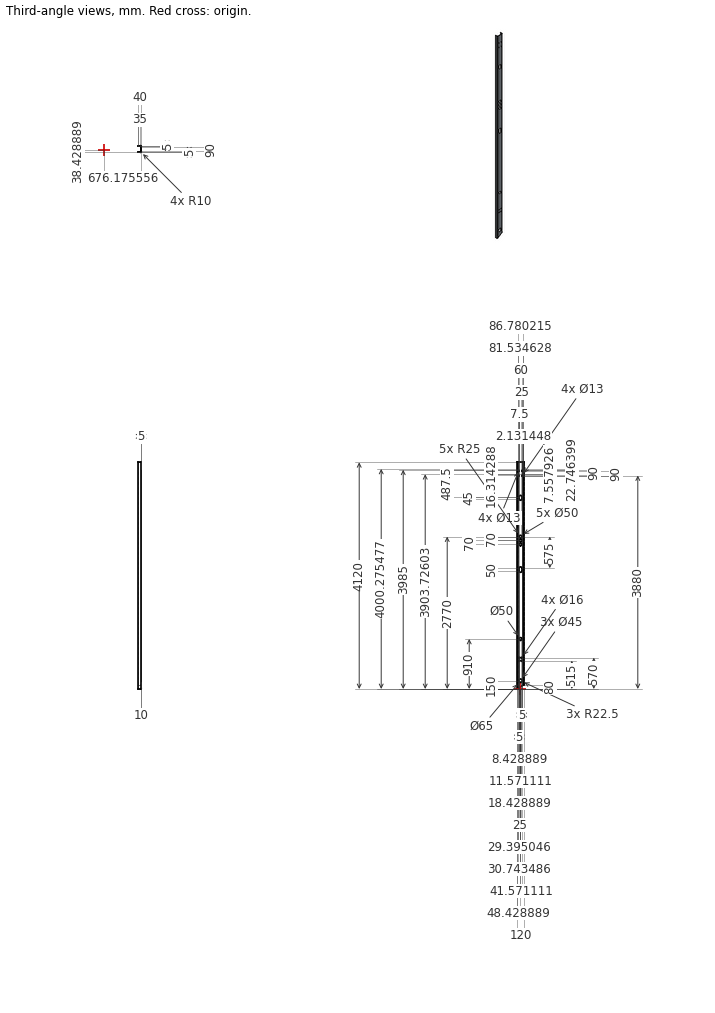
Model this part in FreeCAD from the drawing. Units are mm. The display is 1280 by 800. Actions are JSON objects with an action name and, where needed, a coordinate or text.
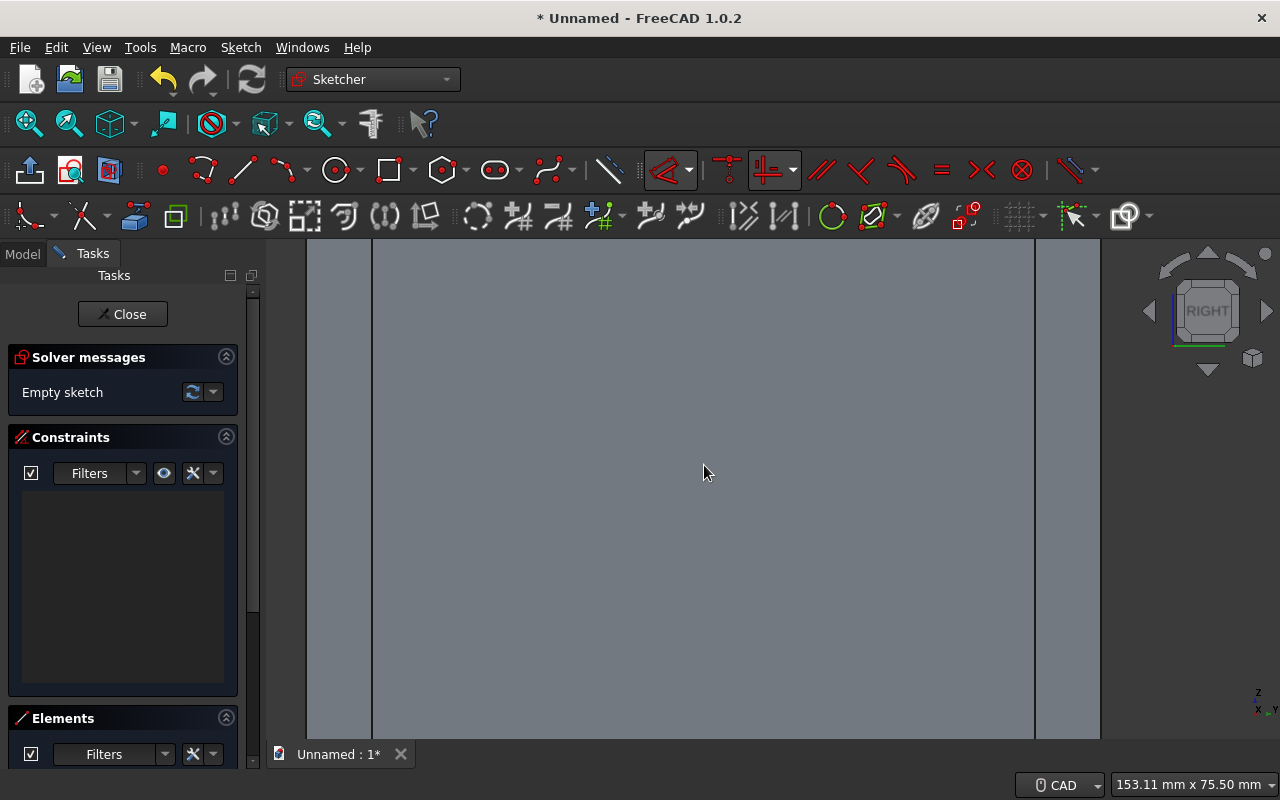
{"action": "left_click", "coordinate": [336, 170]}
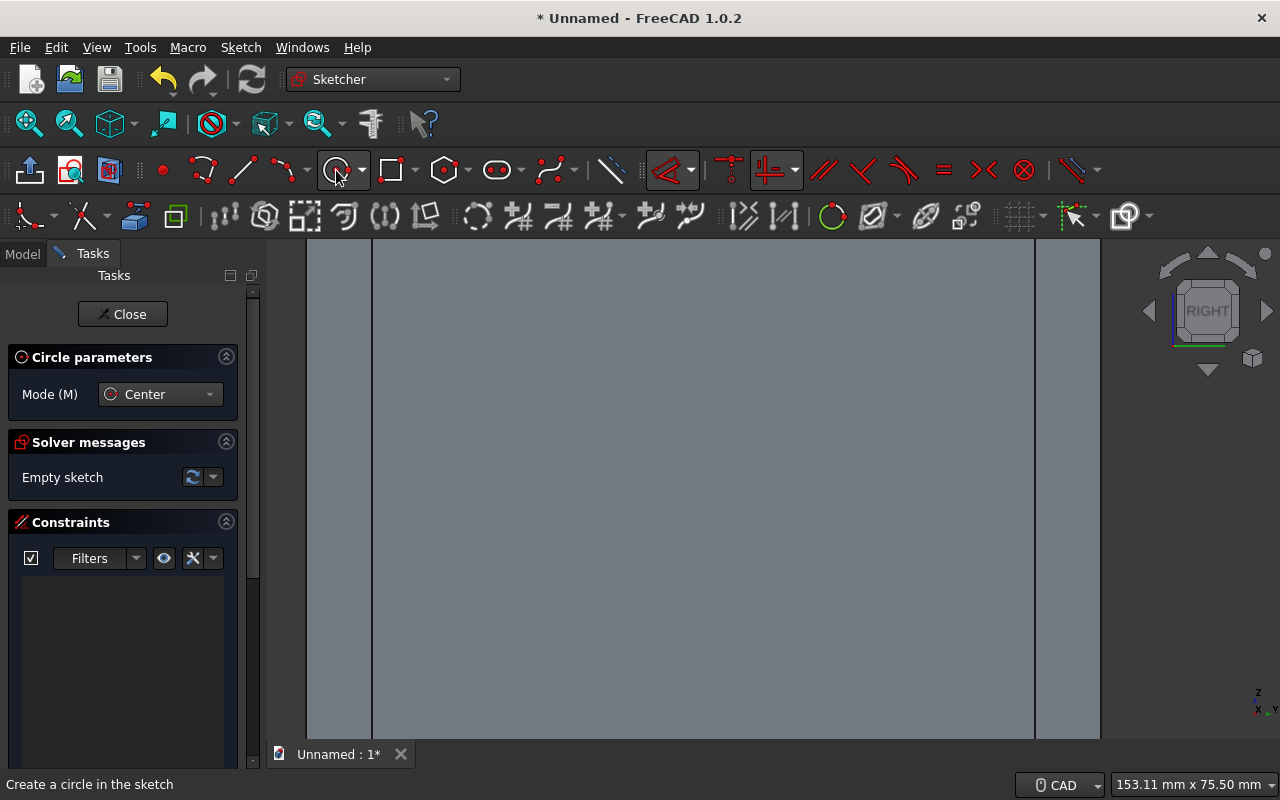
{"action": "left_click", "coordinate": [703, 488]}
{"action": "mouse_move", "coordinate": [821, 370]}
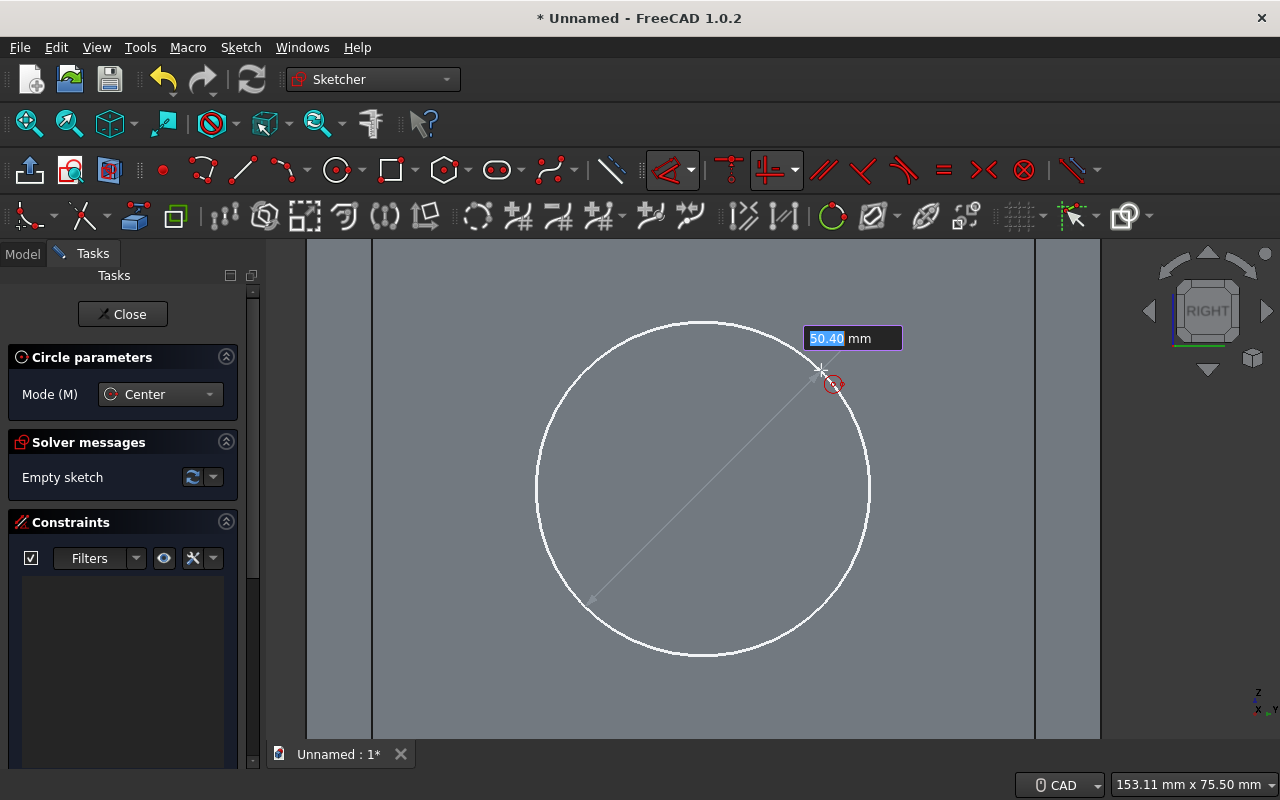
{"action": "type", "text": "50"}
{"action": "key", "text": "Return"}
{"action": "key", "text": "Escape"}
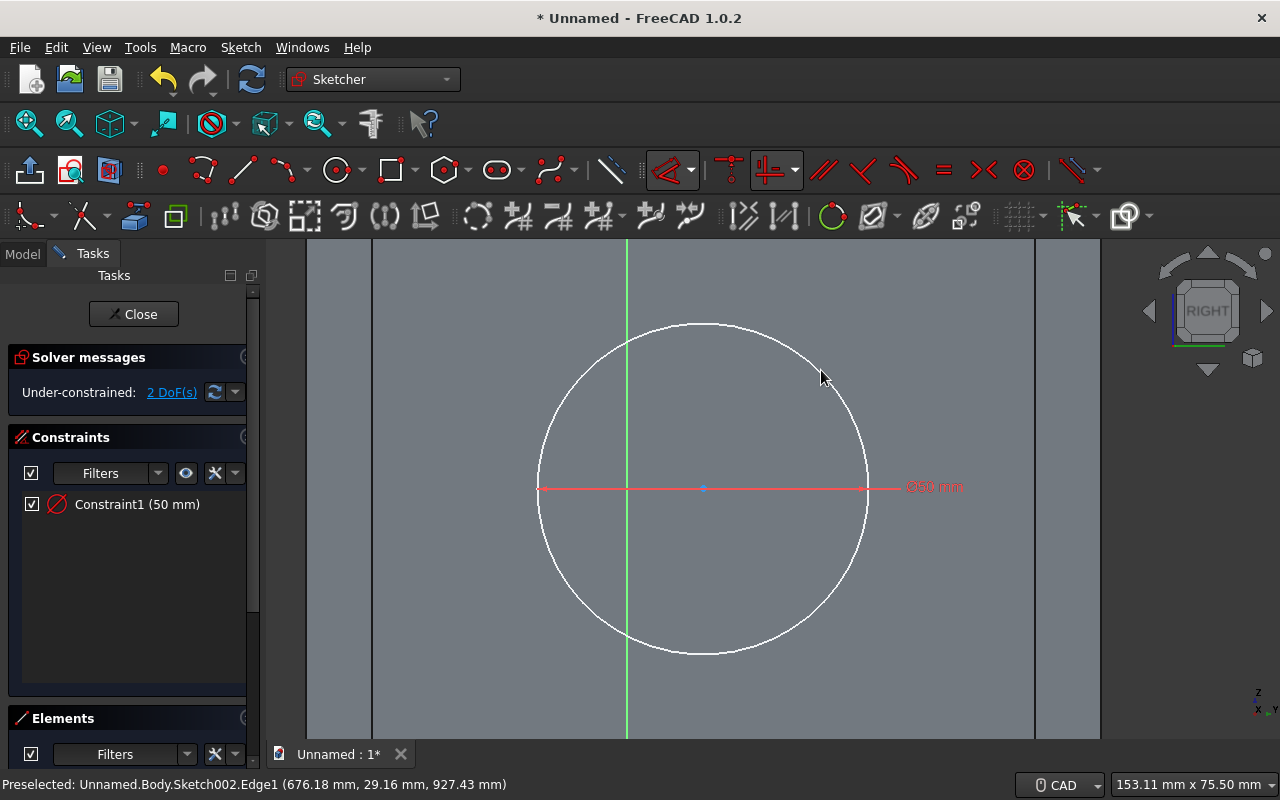
{"action": "left_click", "coordinate": [703, 489]}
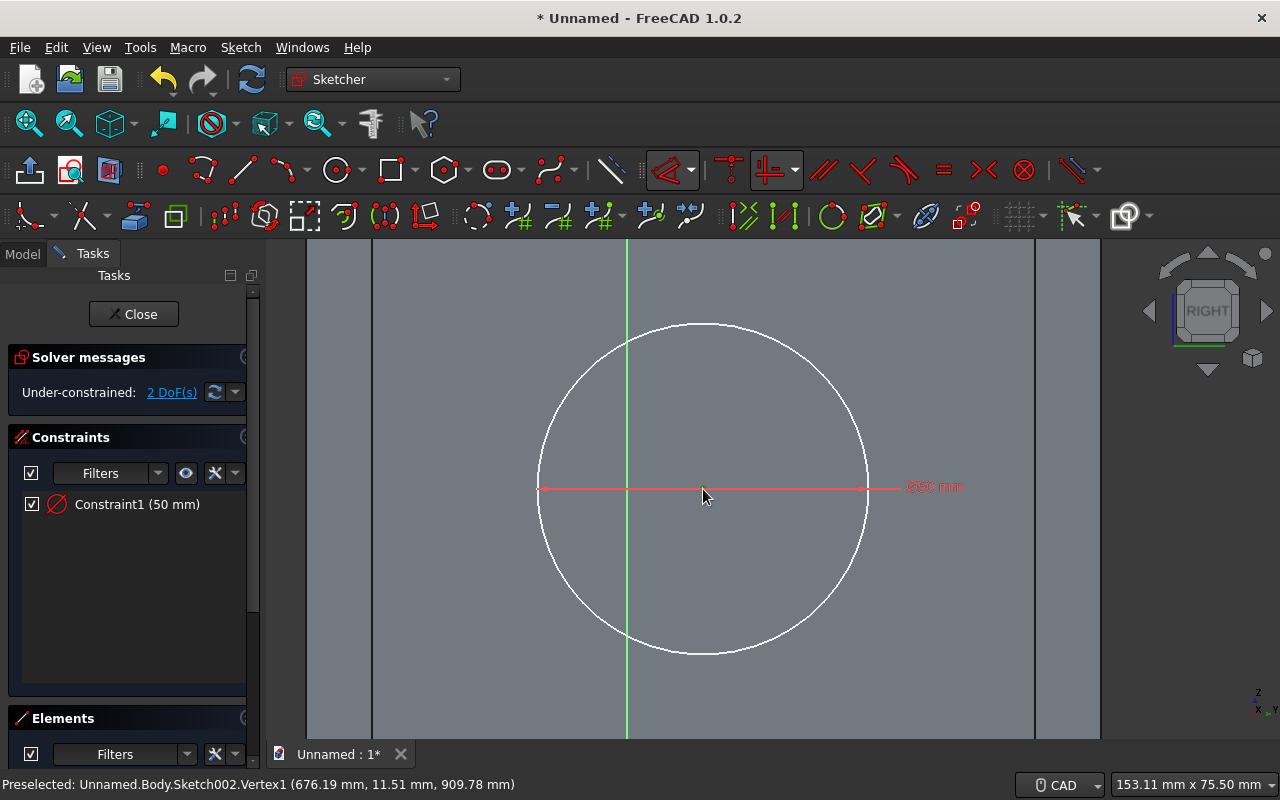
{"action": "key", "text": "i"}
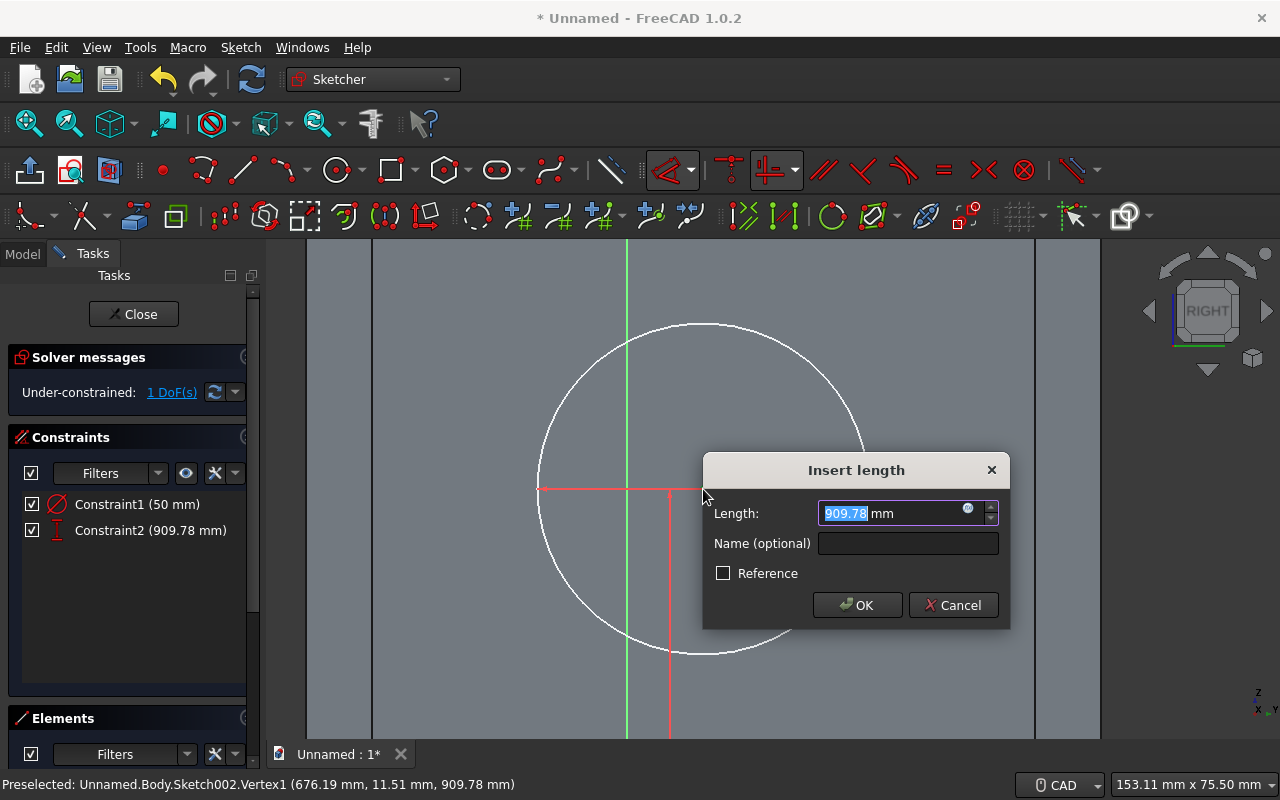
{"action": "type", "text": "910"}
{"action": "key", "text": "Return"}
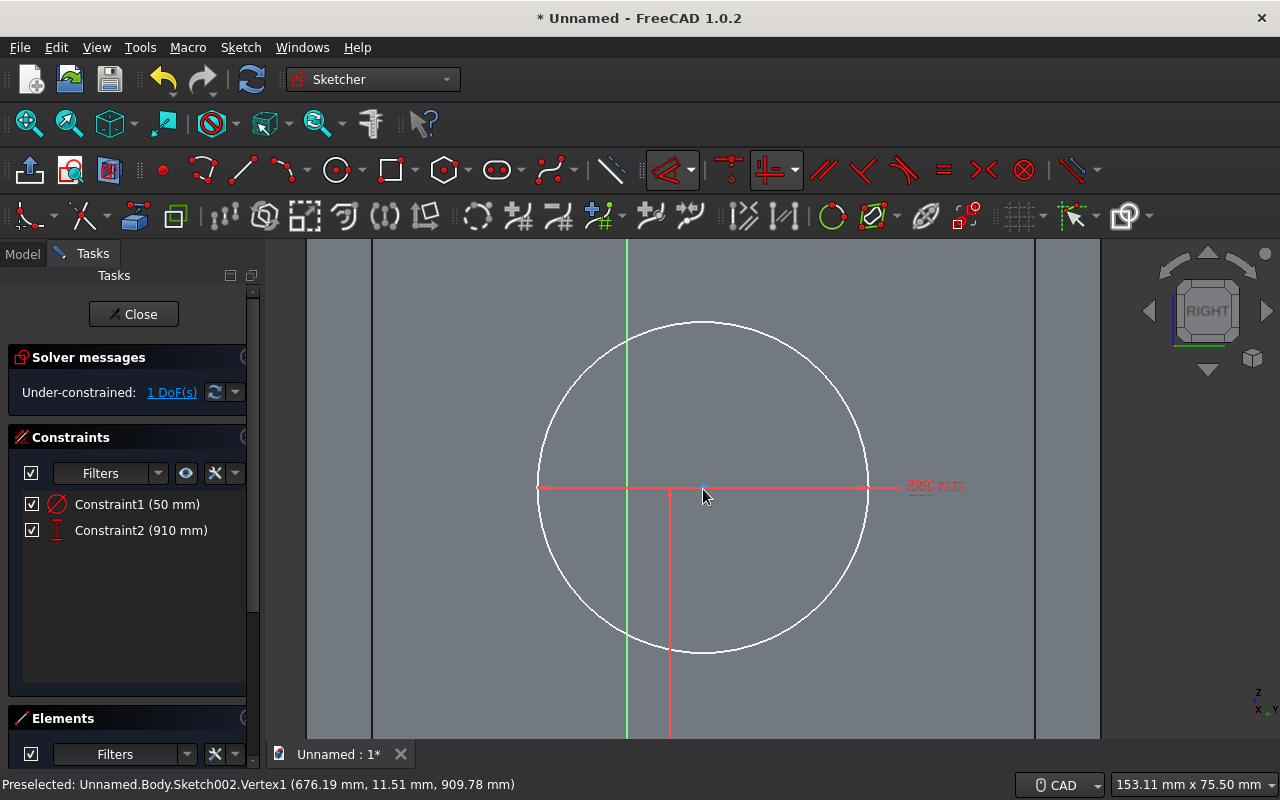
{"action": "left_click", "coordinate": [703, 488]}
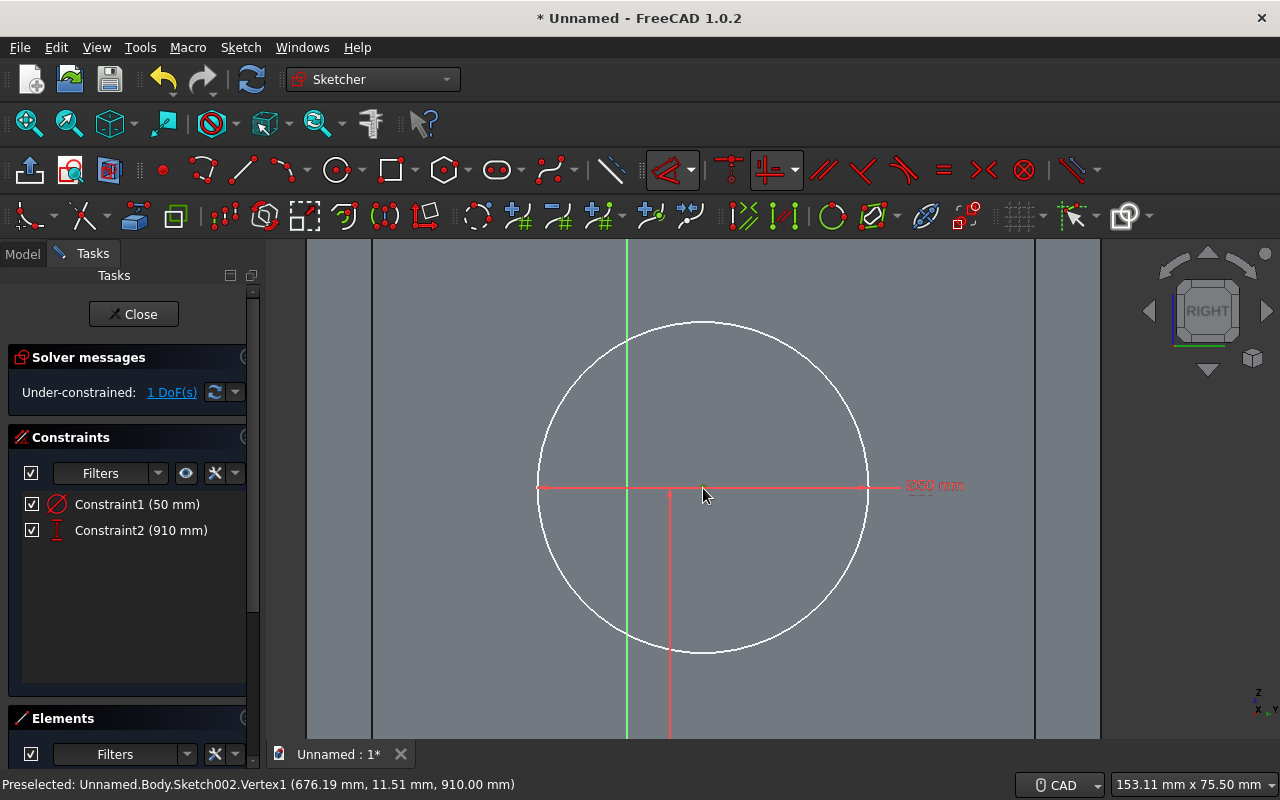
{"action": "left_click", "coordinate": [694, 170]}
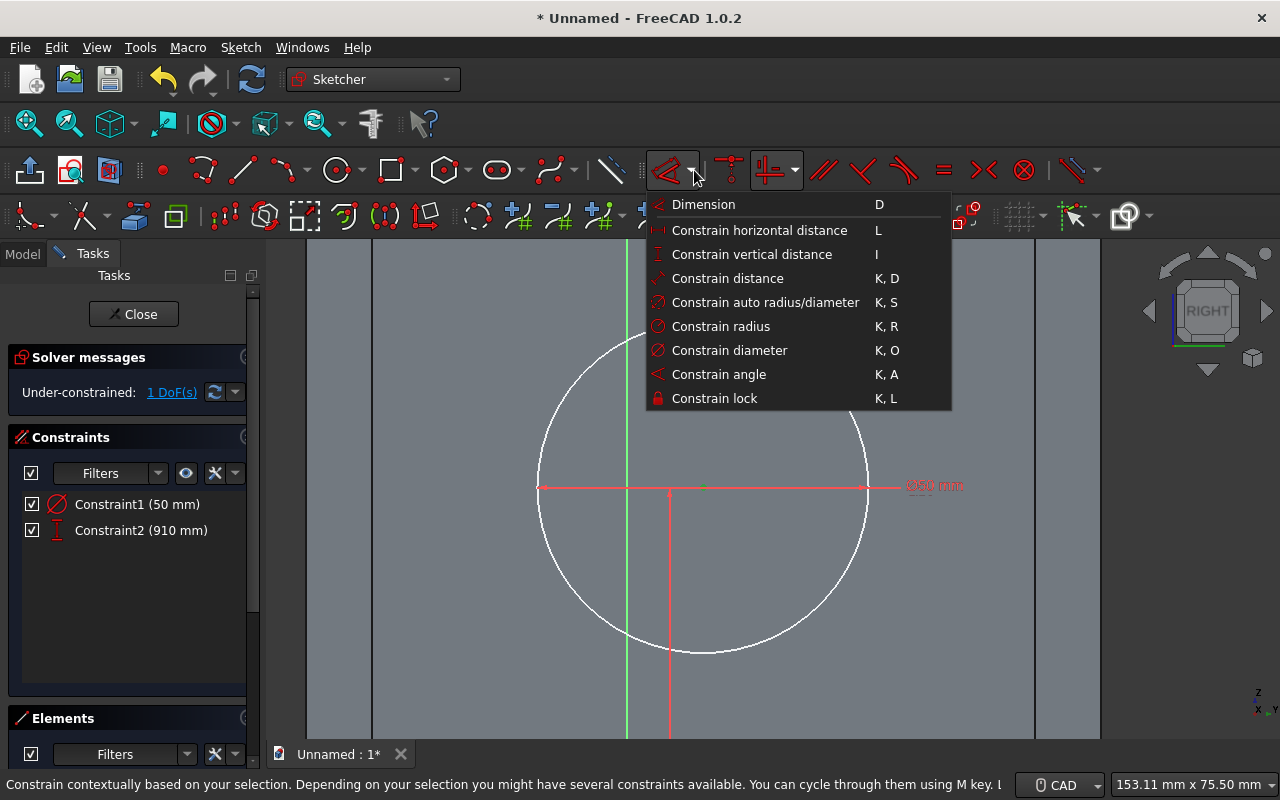
{"action": "left_click", "coordinate": [799, 230]}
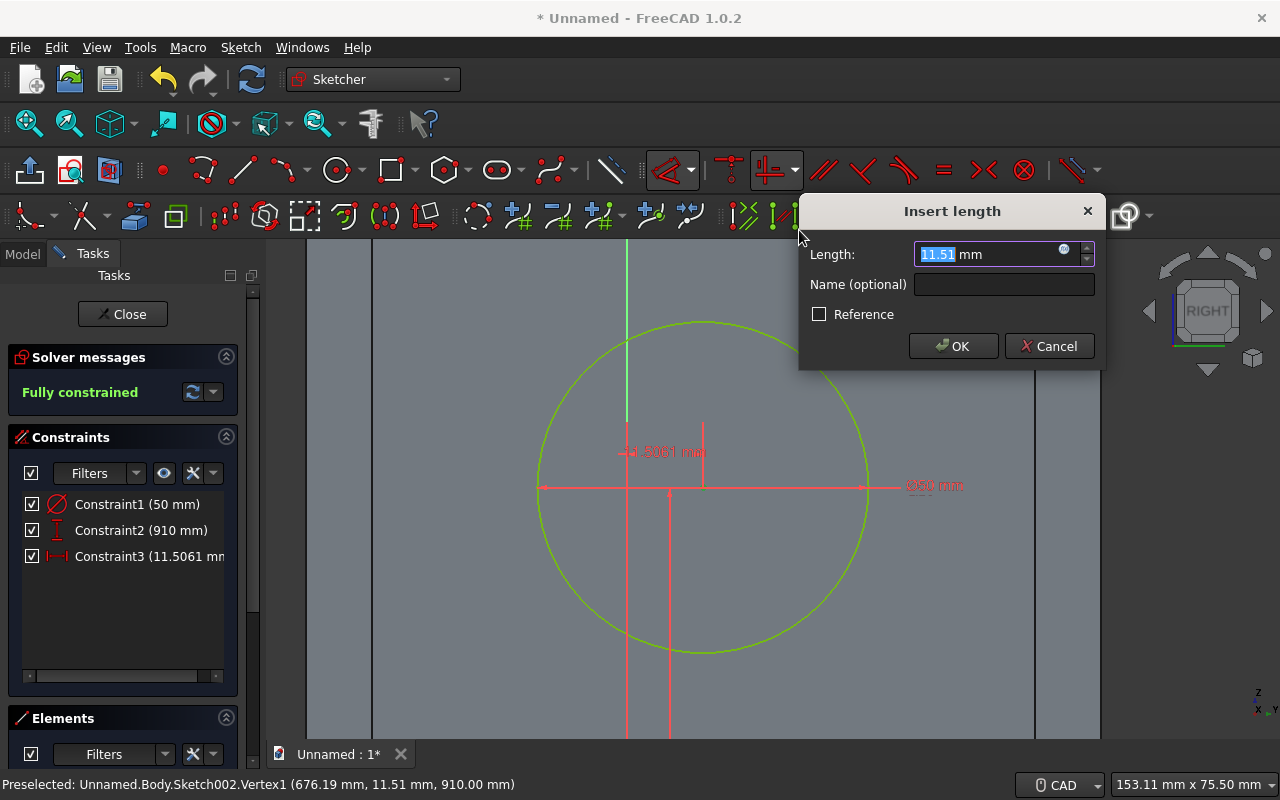
{"action": "type", "text": "11.571111"}
{"action": "key", "text": "Return"}